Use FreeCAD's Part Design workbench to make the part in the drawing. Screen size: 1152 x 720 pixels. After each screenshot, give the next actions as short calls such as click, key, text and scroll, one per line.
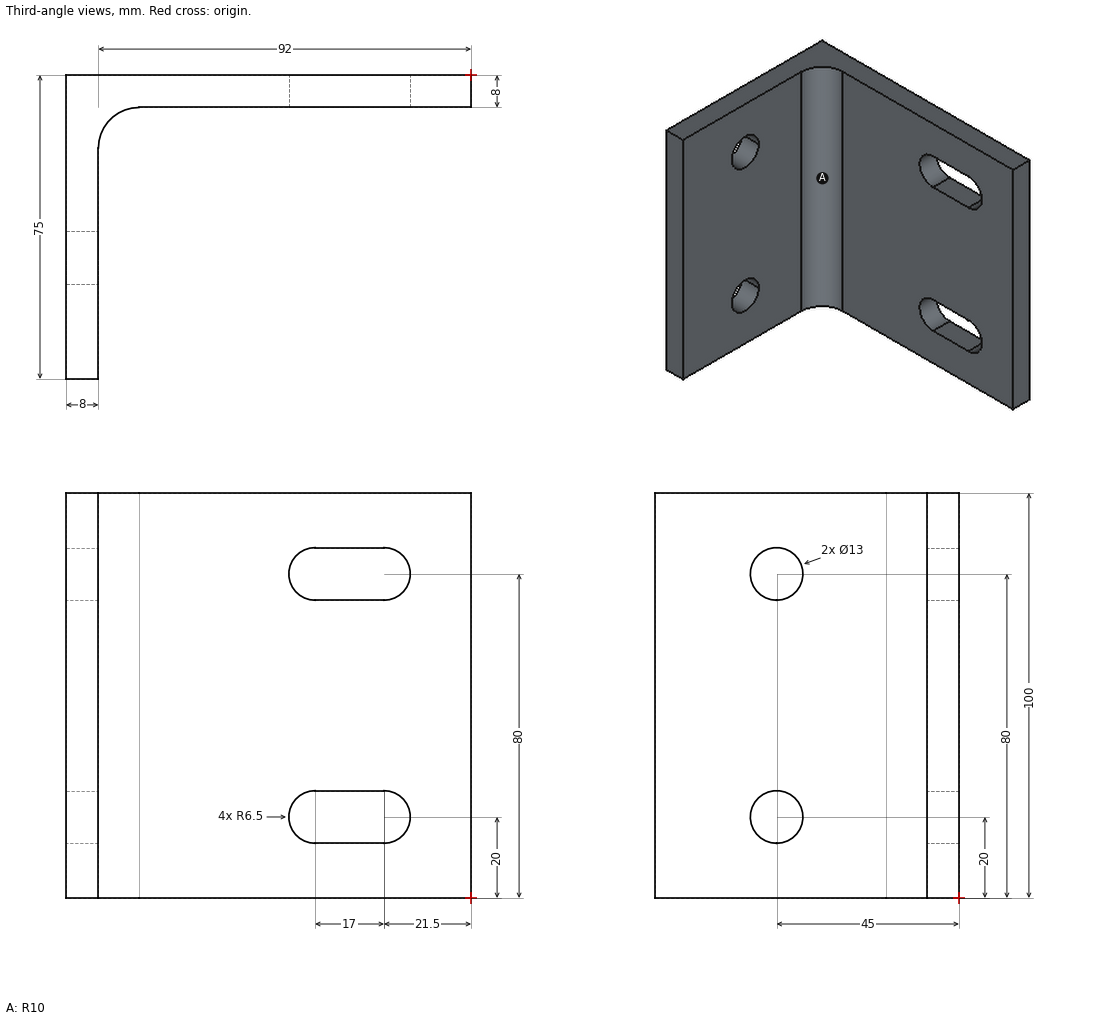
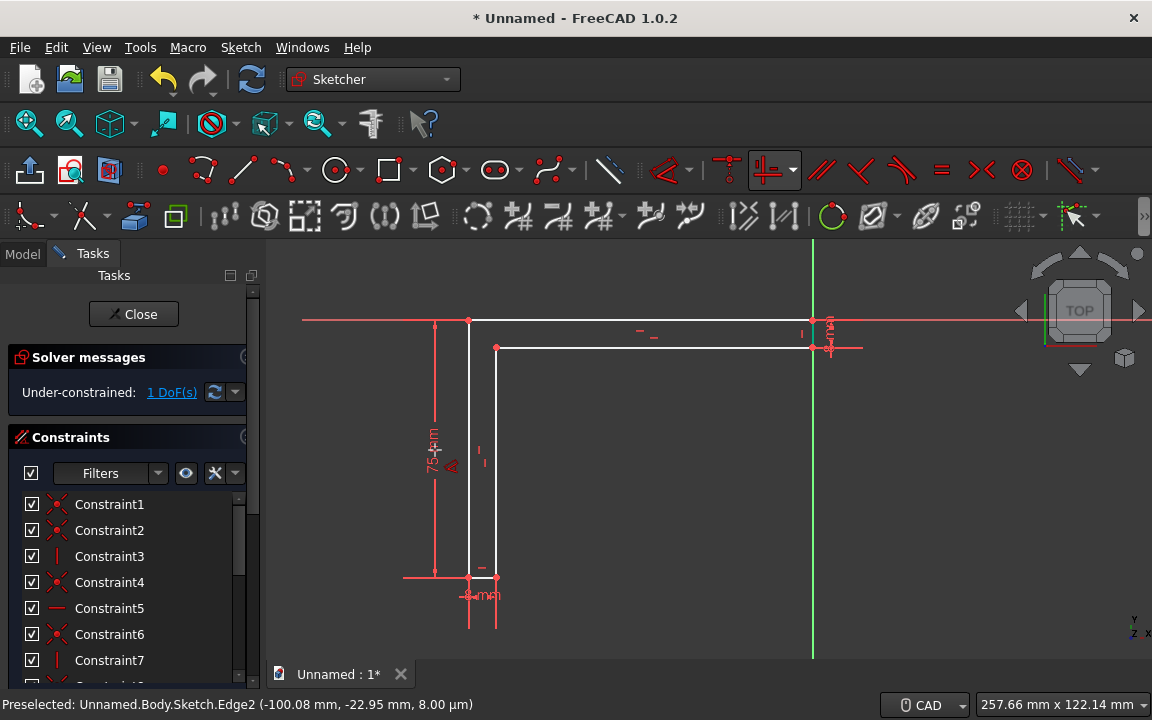
click(591, 348)
click(654, 382)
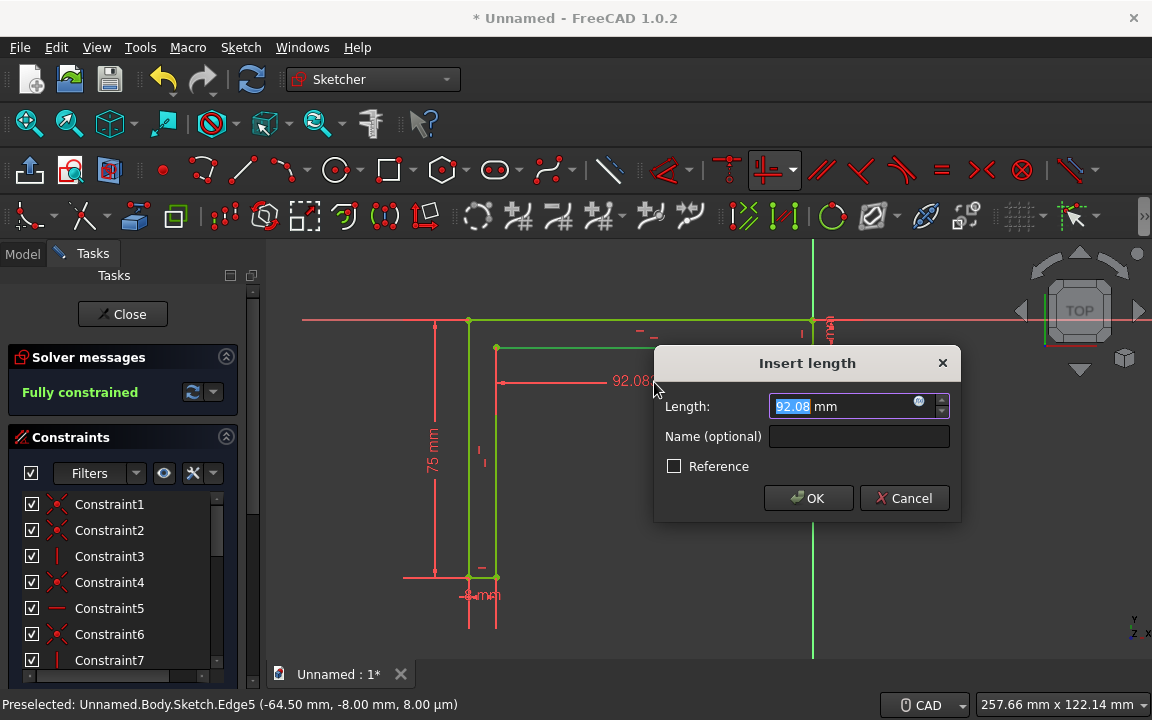
text(92)
key(Return)
key(Escape)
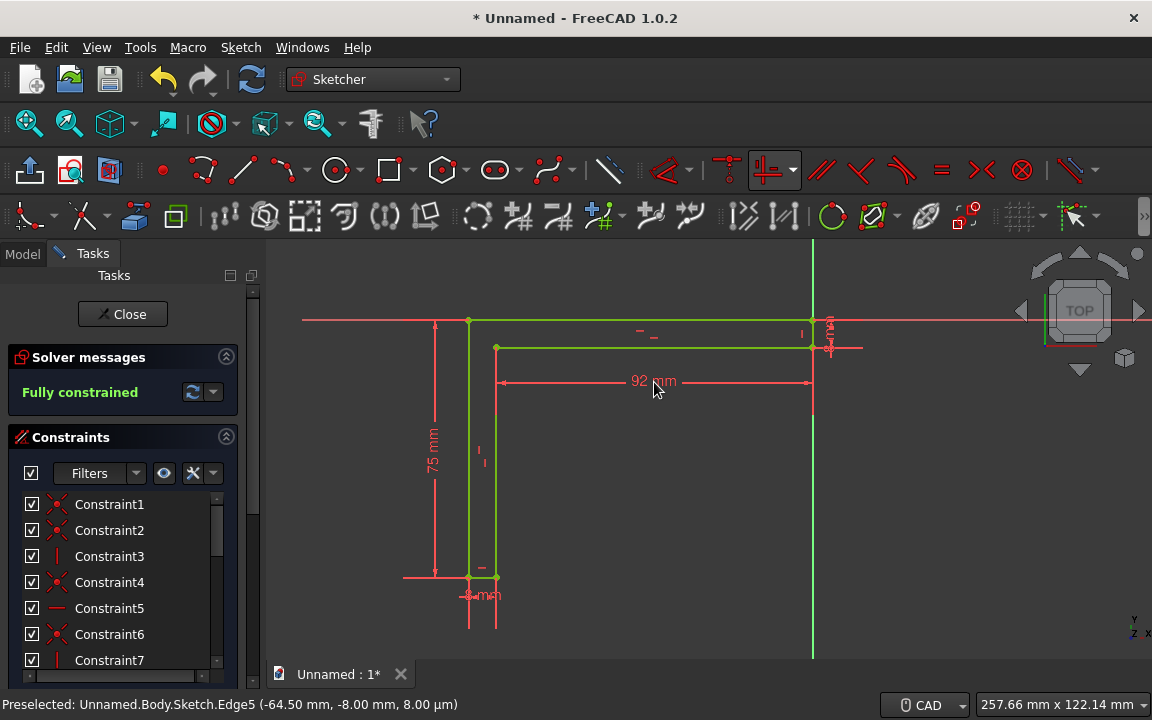
click(123, 314)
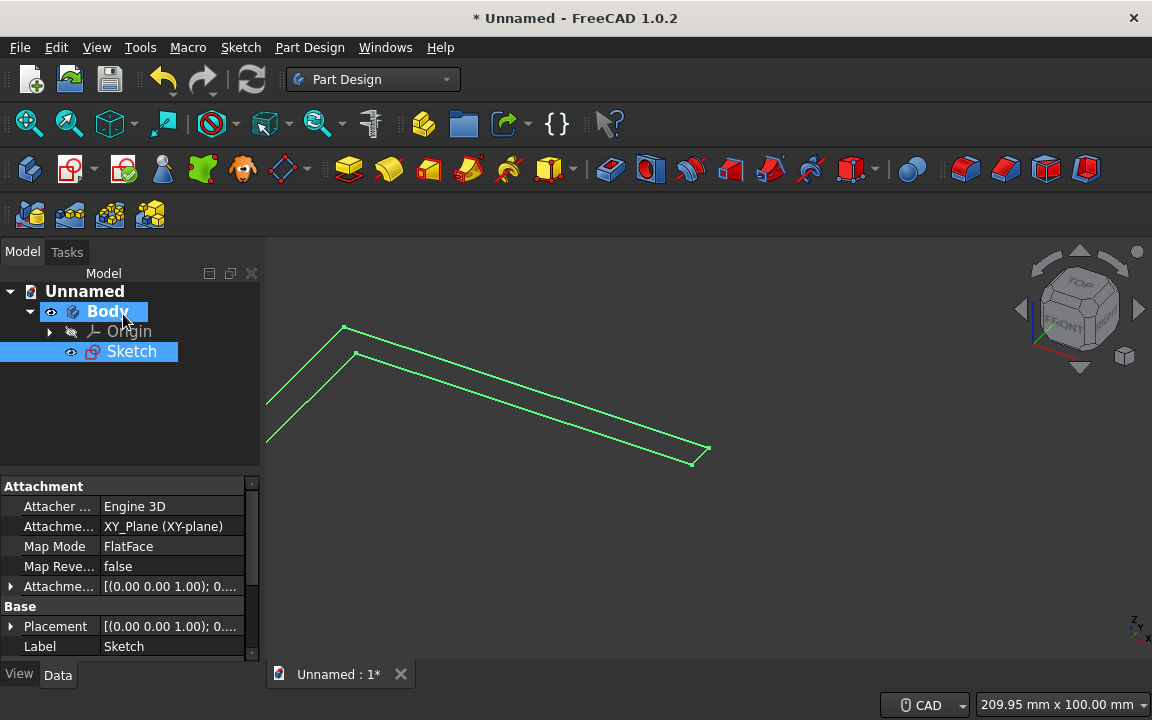
click(350, 170)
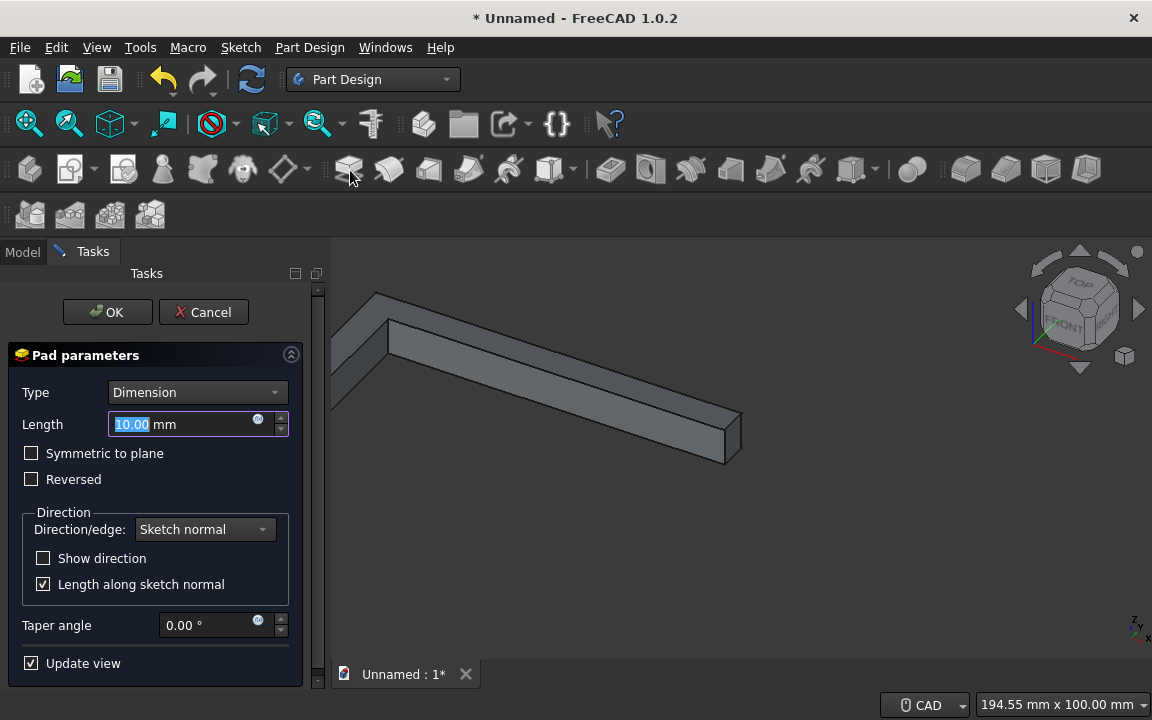
text(100)
key(Tab)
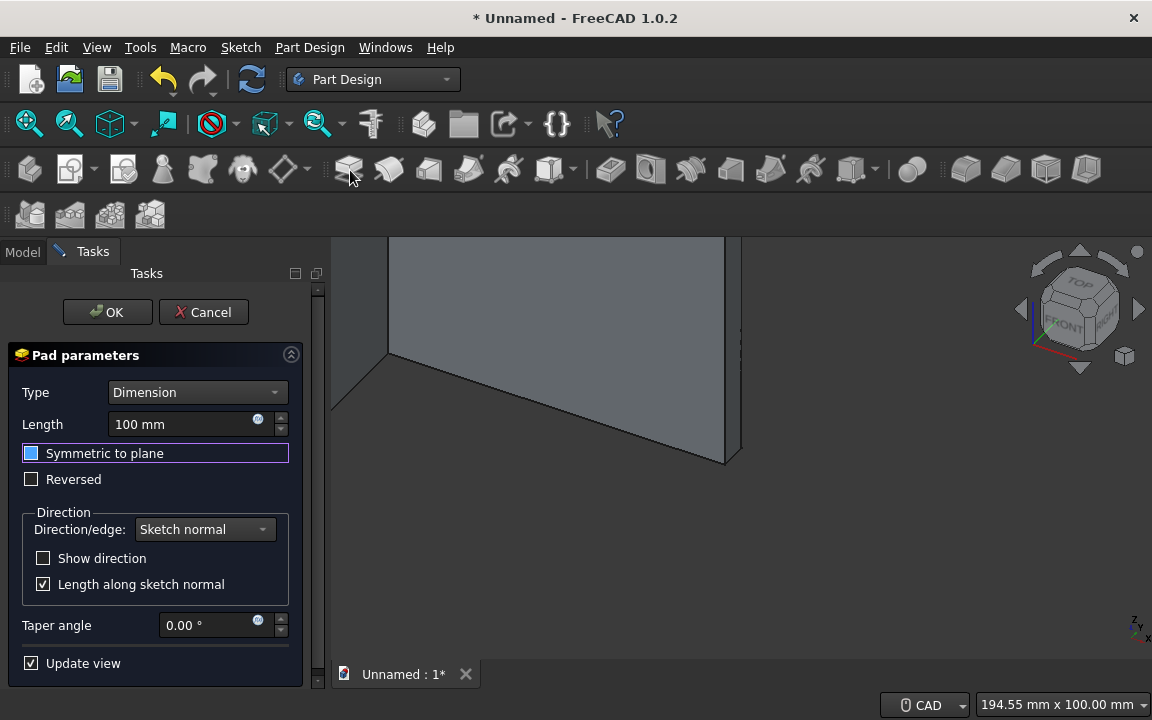
click(108, 312)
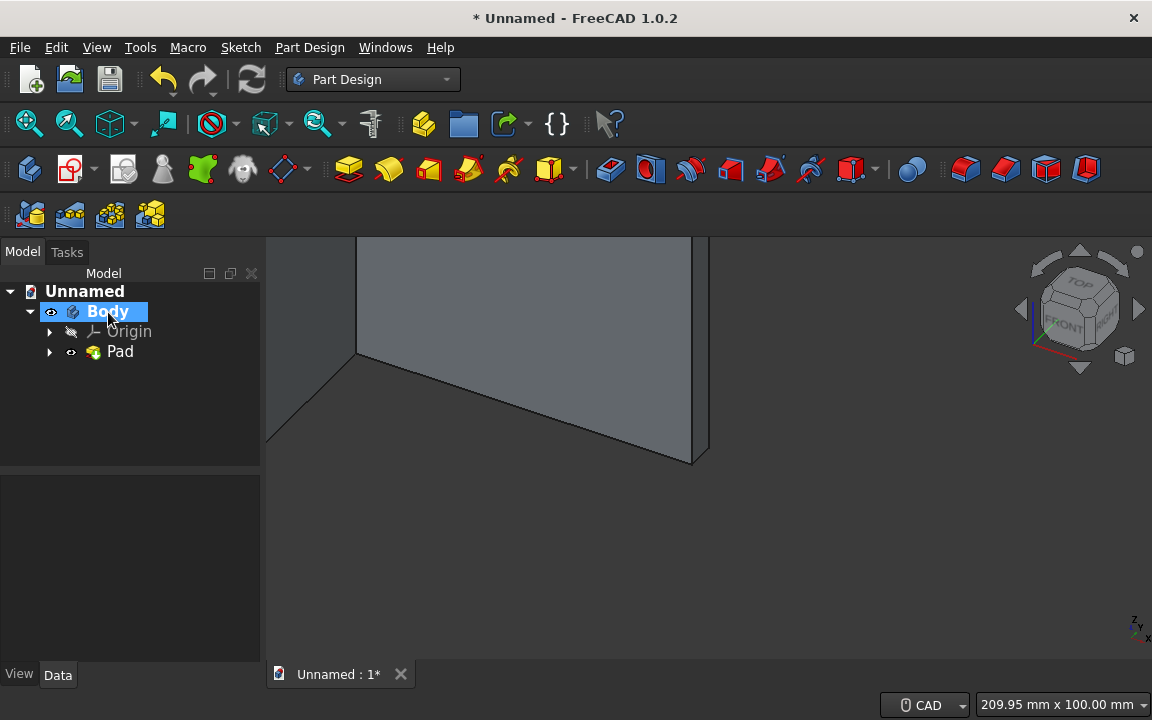
click(30, 124)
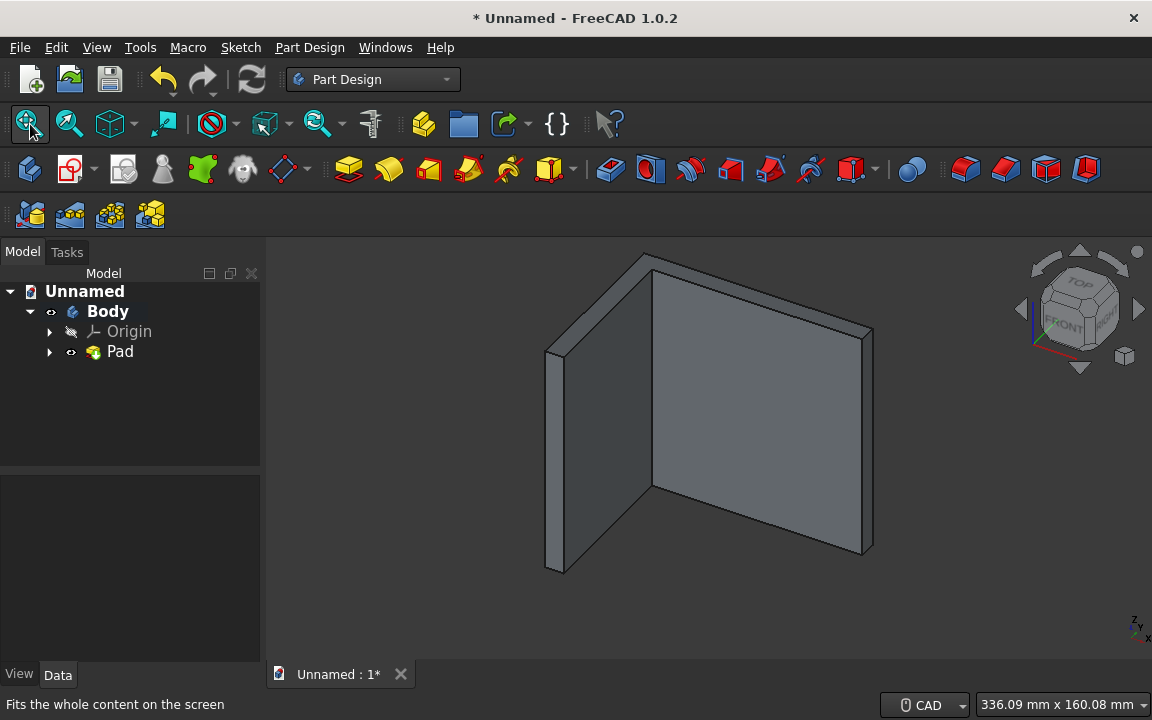
key(4)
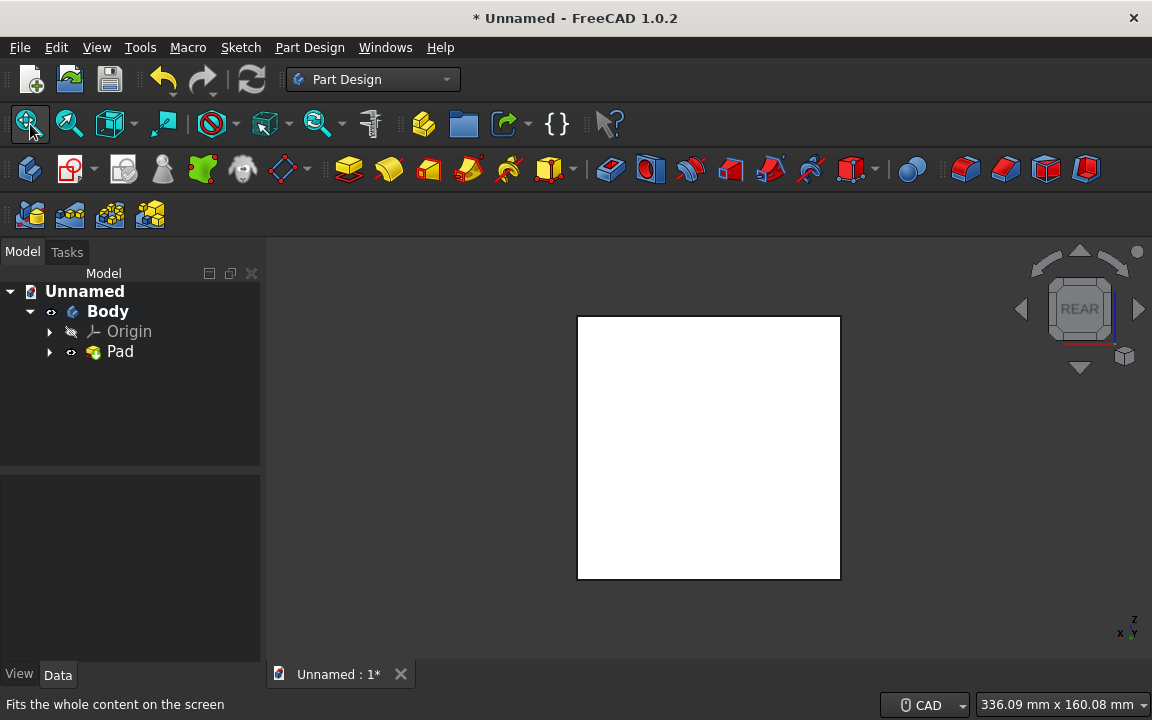
click(709, 447)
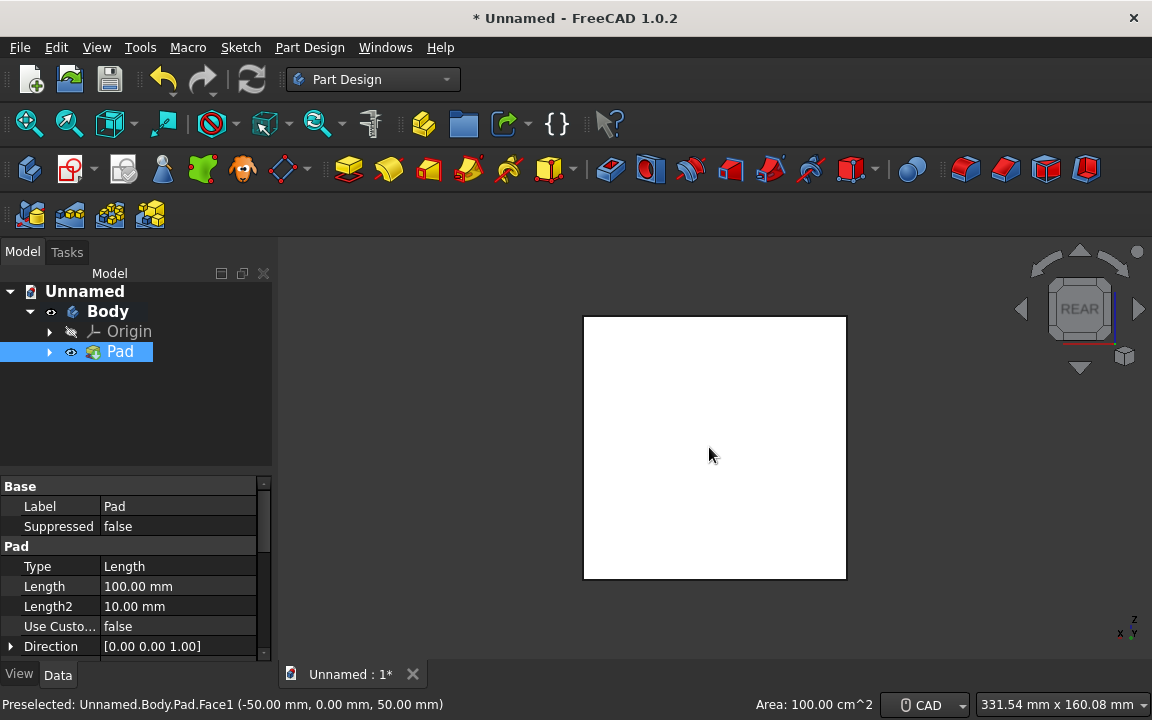
click(70, 170)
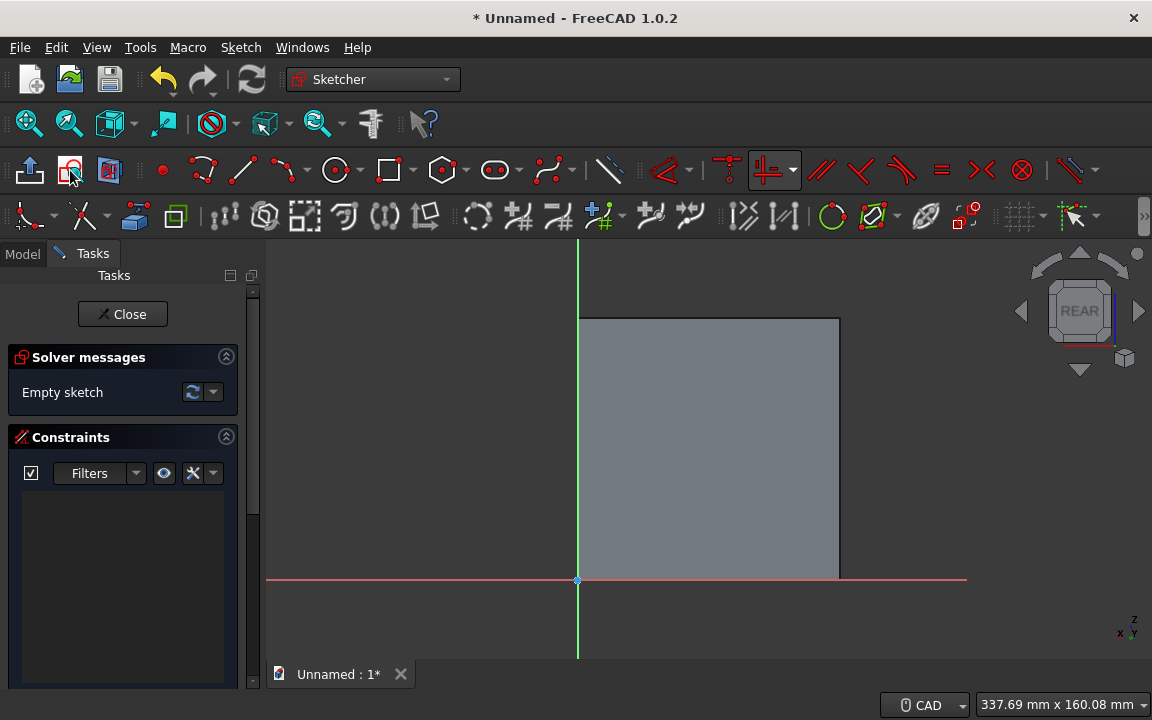
click(496, 170)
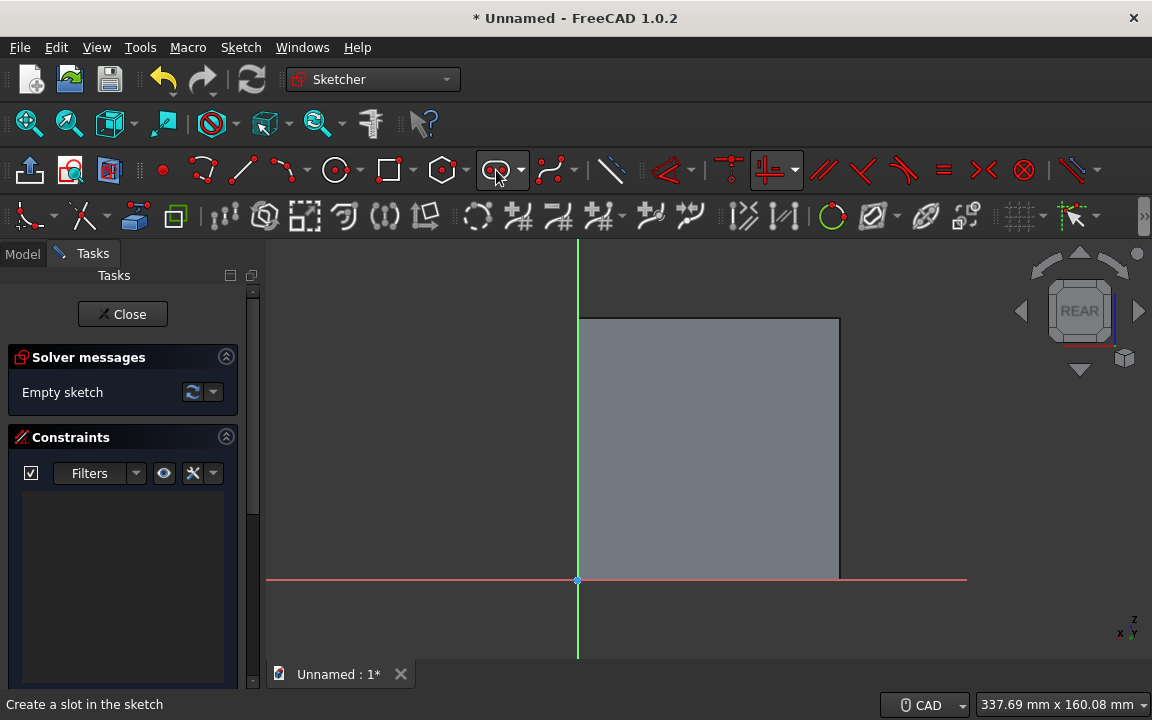
scroll(634, 528, up, 2)